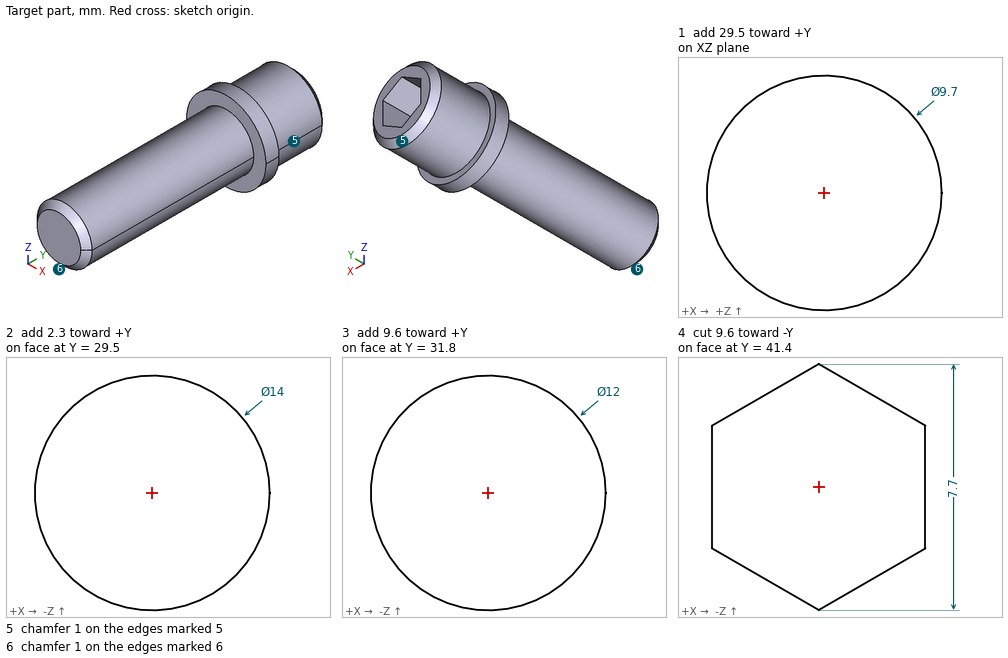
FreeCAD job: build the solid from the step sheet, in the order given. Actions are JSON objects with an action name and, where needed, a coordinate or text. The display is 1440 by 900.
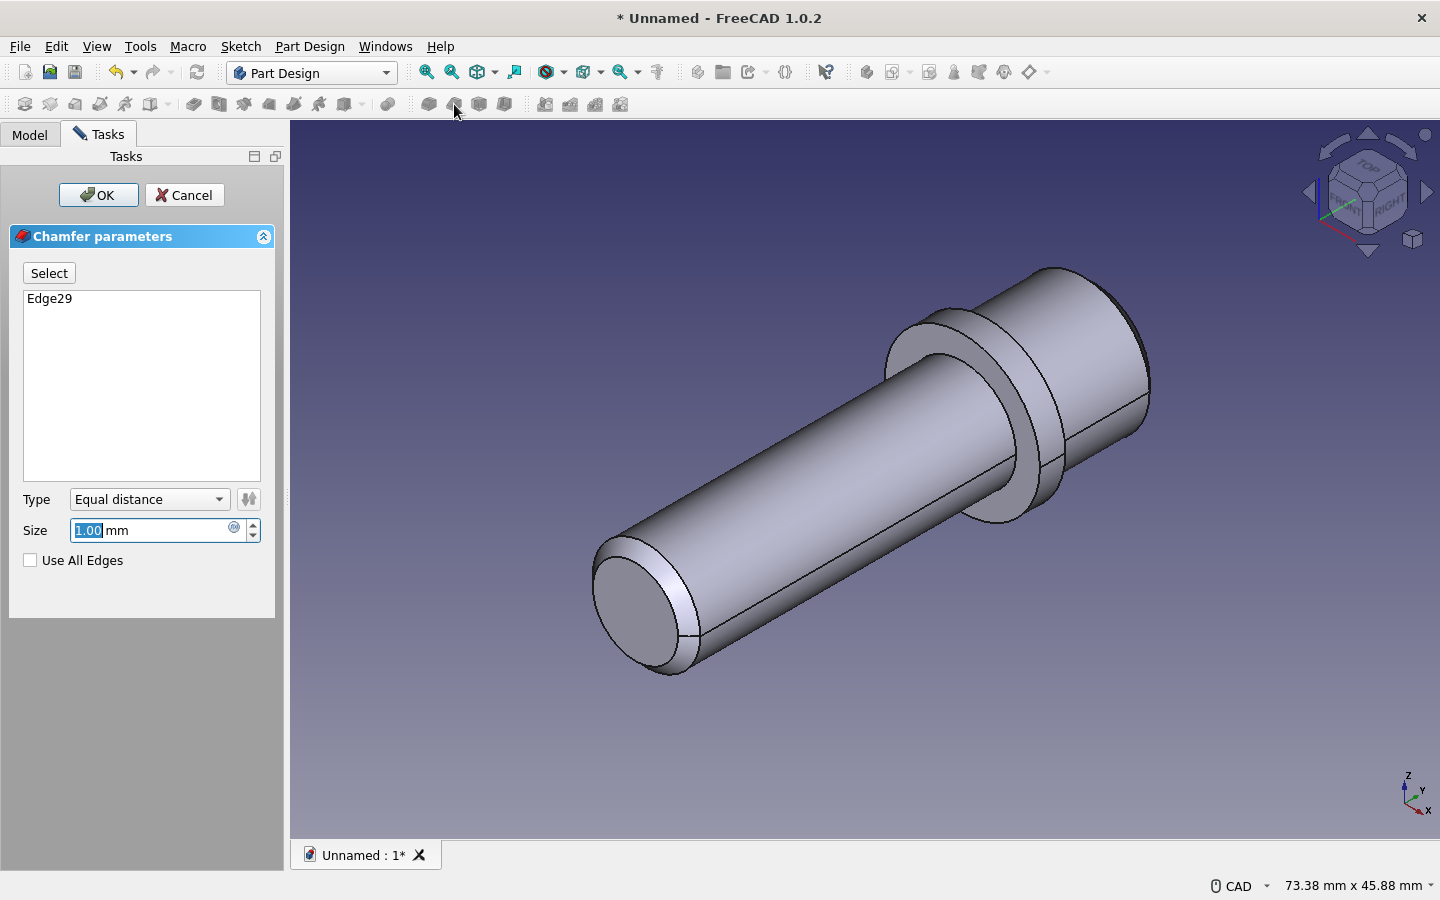
{"action": "type", "text": "1"}
{"action": "key", "text": "Tab"}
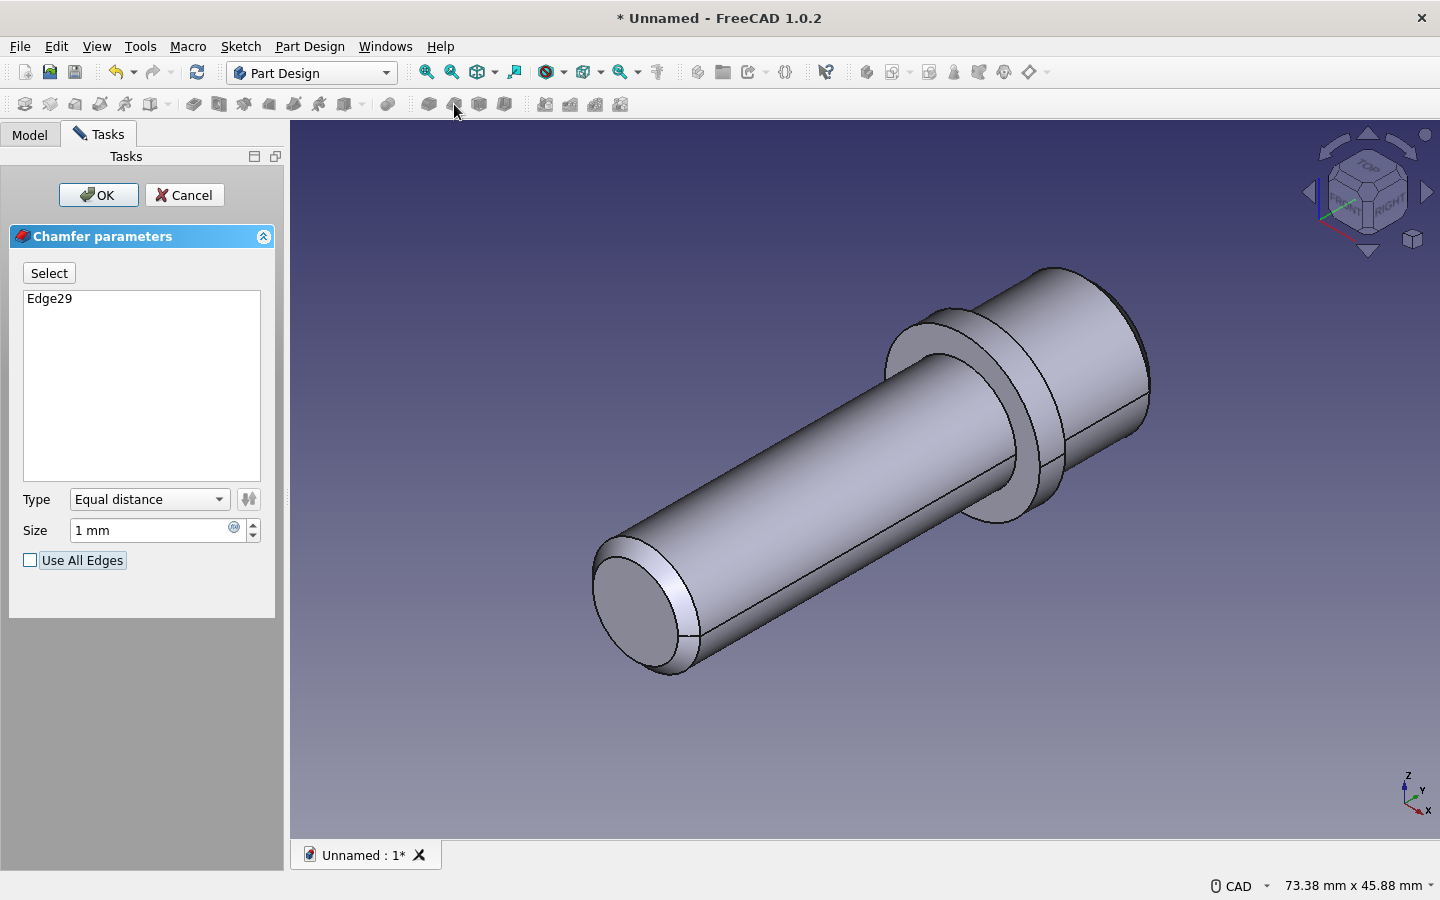
{"action": "left_click", "coordinate": [99, 195]}